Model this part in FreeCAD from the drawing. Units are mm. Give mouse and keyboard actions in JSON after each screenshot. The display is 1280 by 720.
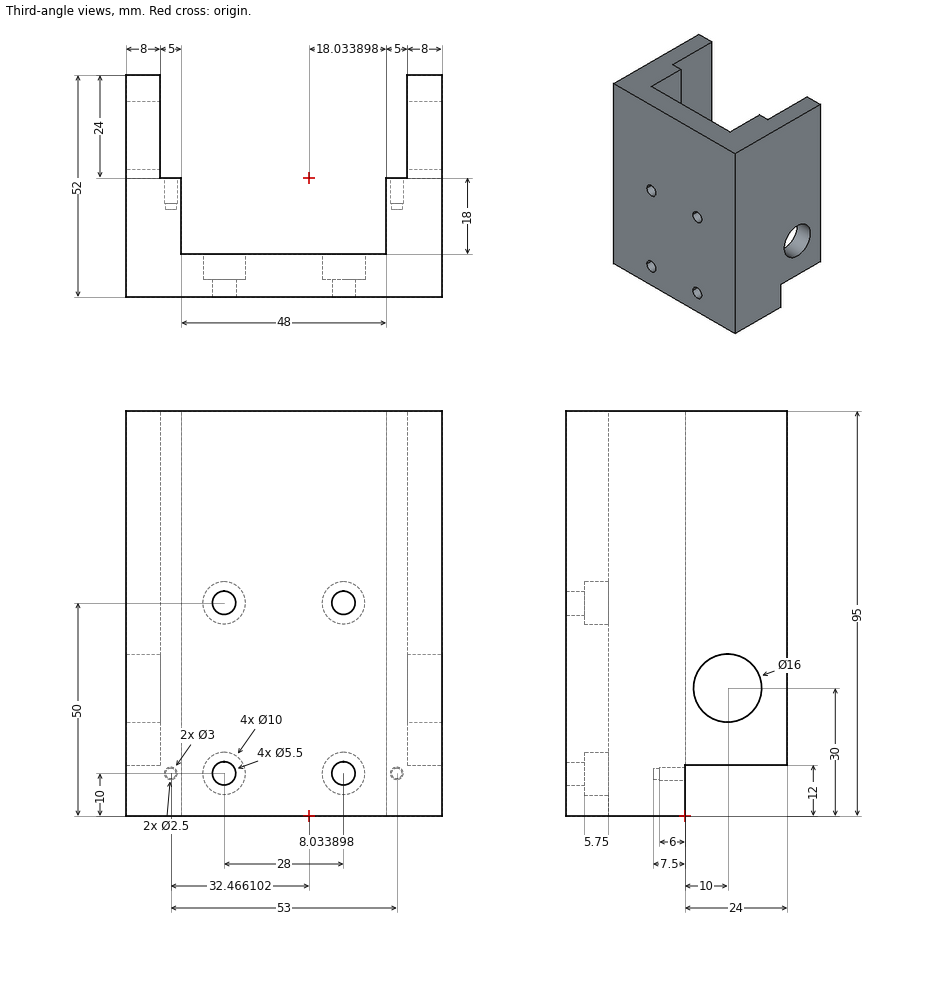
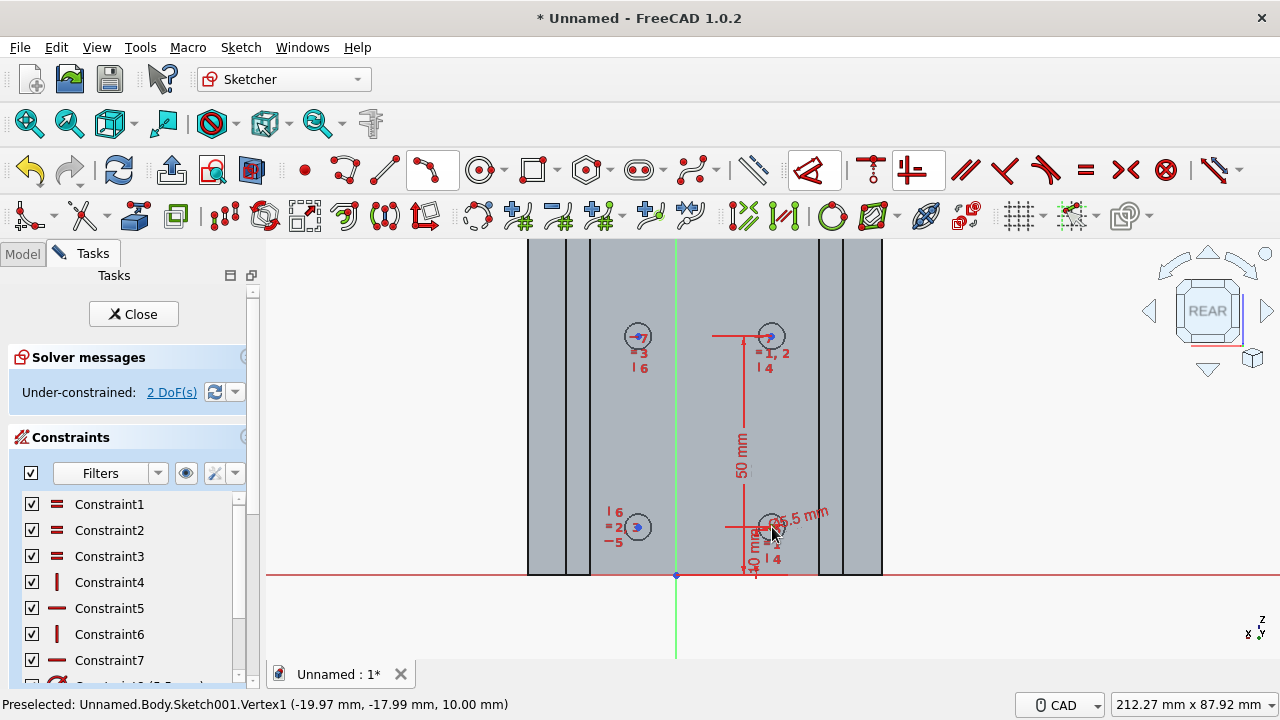
{"action": "left_click", "coordinate": [638, 527]}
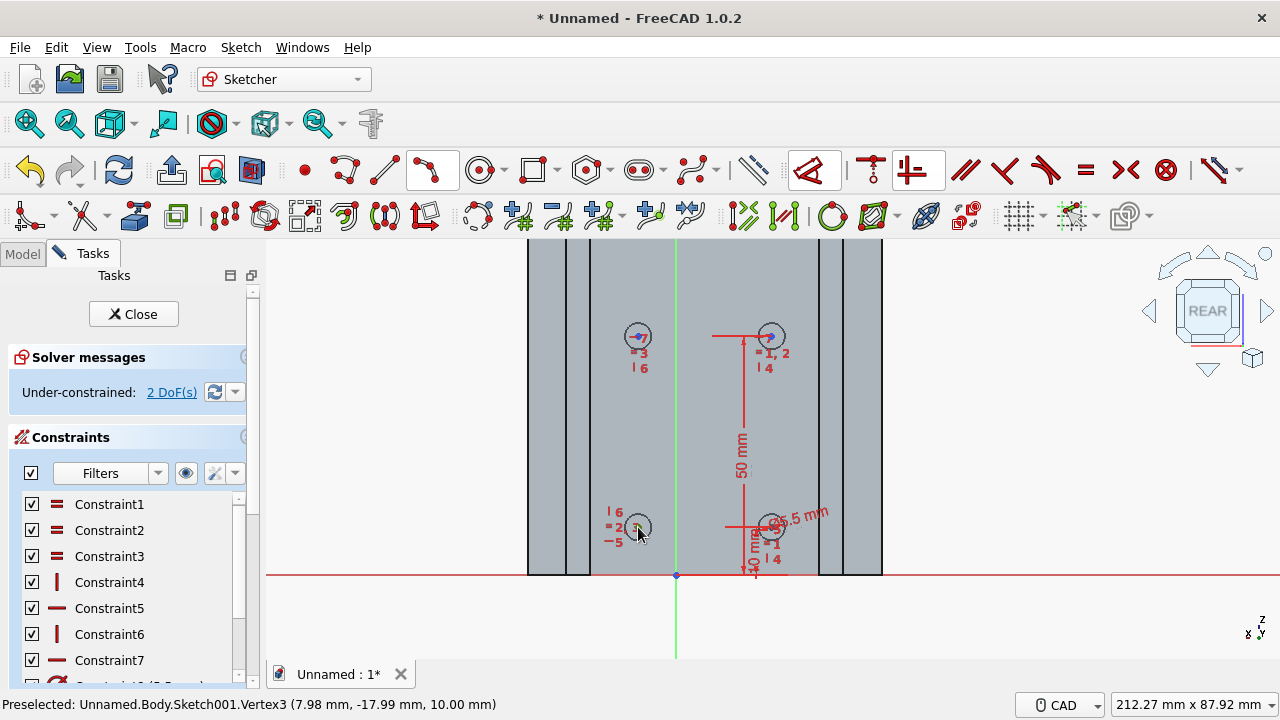
{"action": "key", "text": "l"}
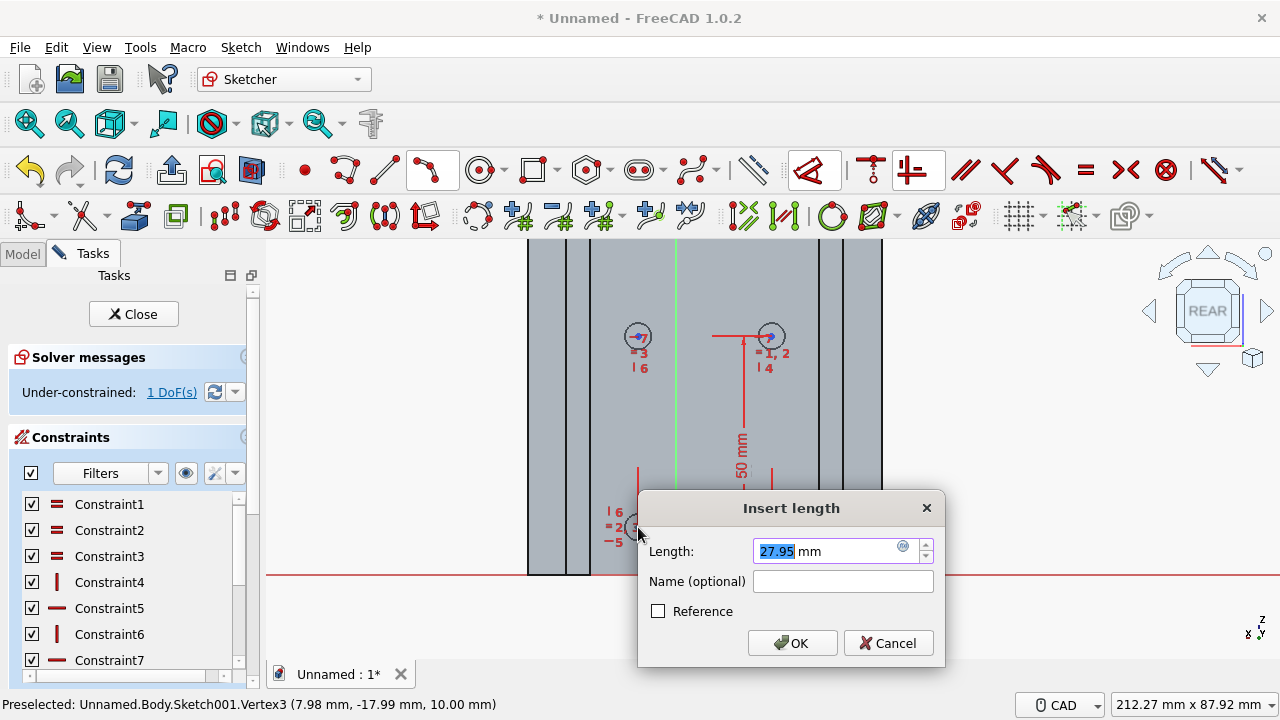
{"action": "type", "text": "28"}
{"action": "key", "text": "Return"}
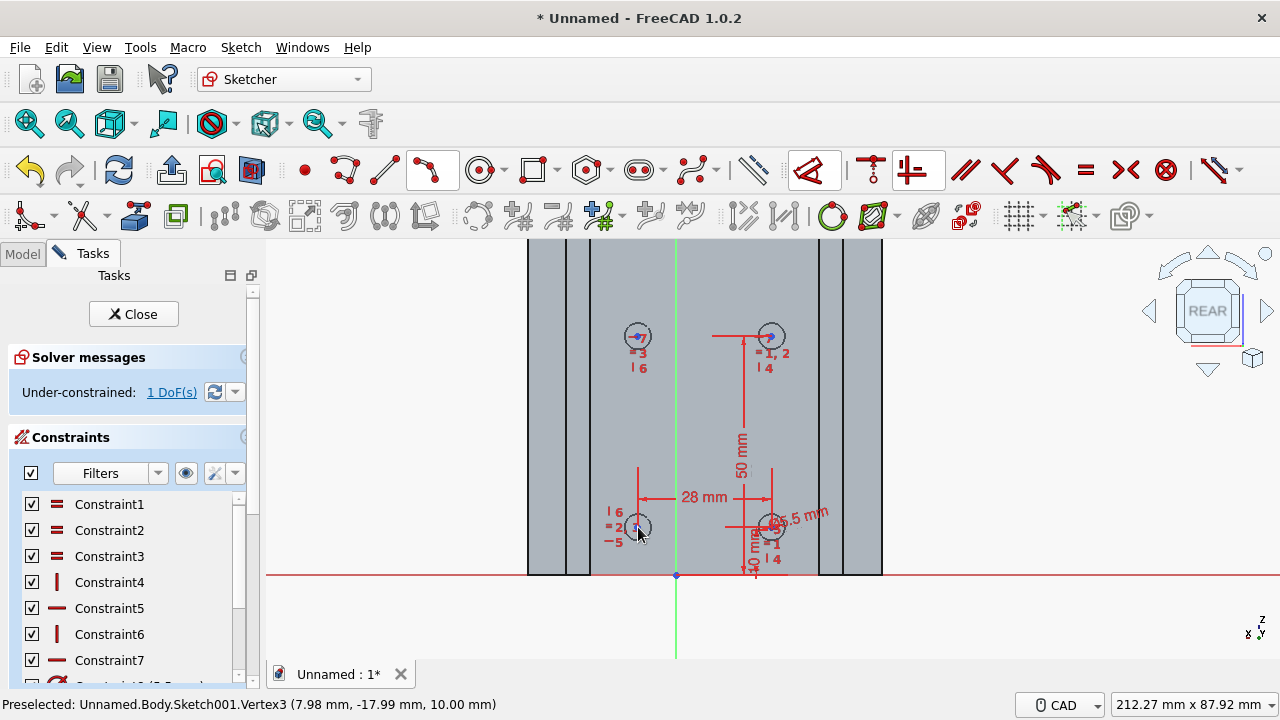
{"action": "left_click", "coordinate": [638, 527]}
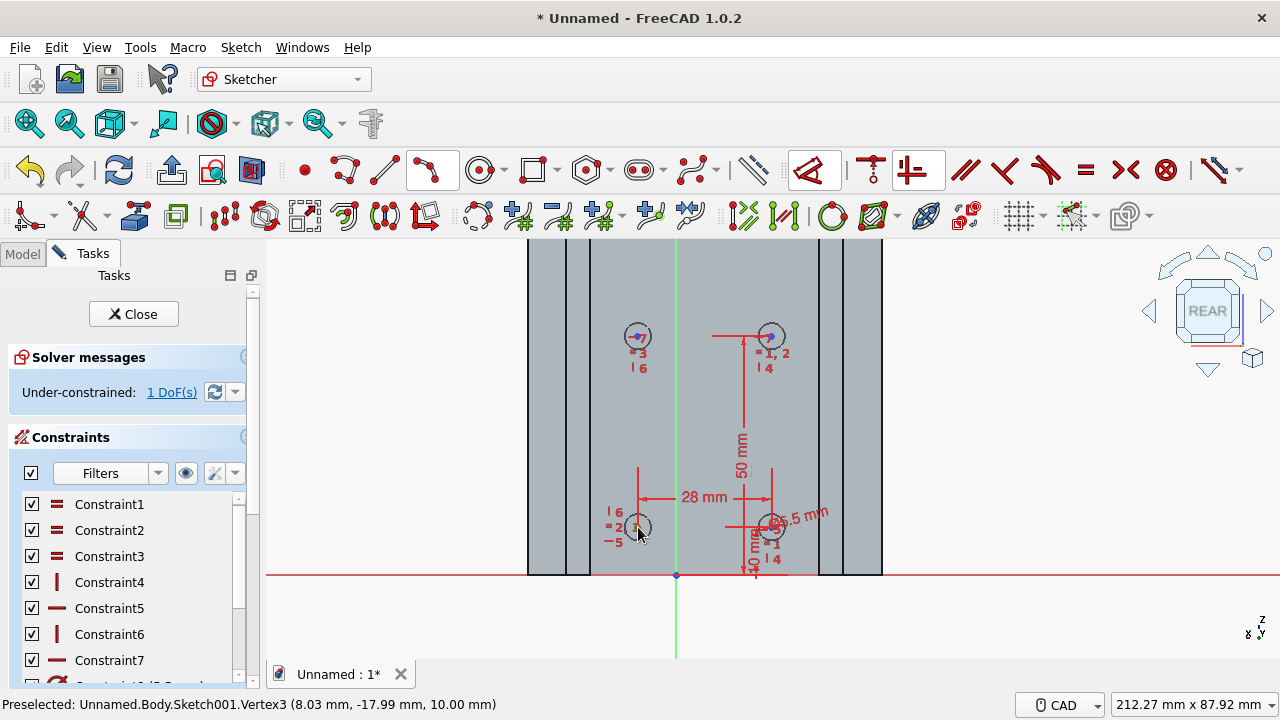
{"action": "key", "text": "l"}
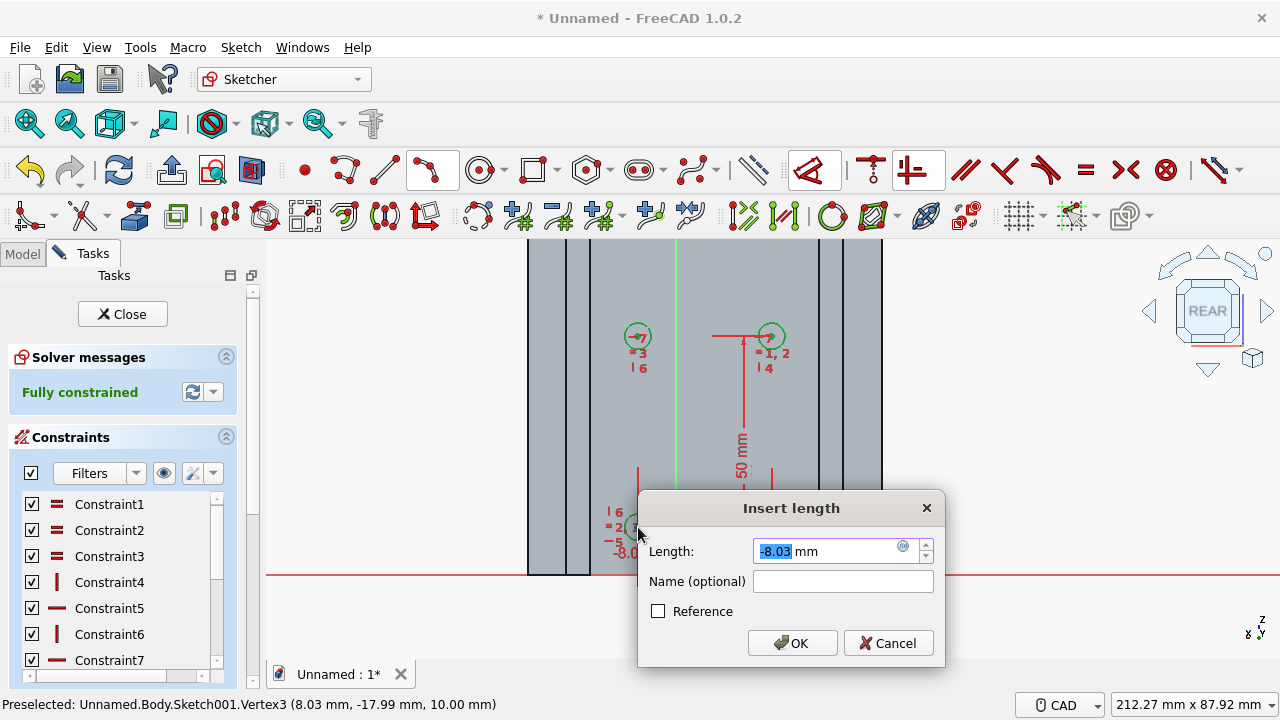
{"action": "type", "text": "-8.033898"}
{"action": "key", "text": "Return"}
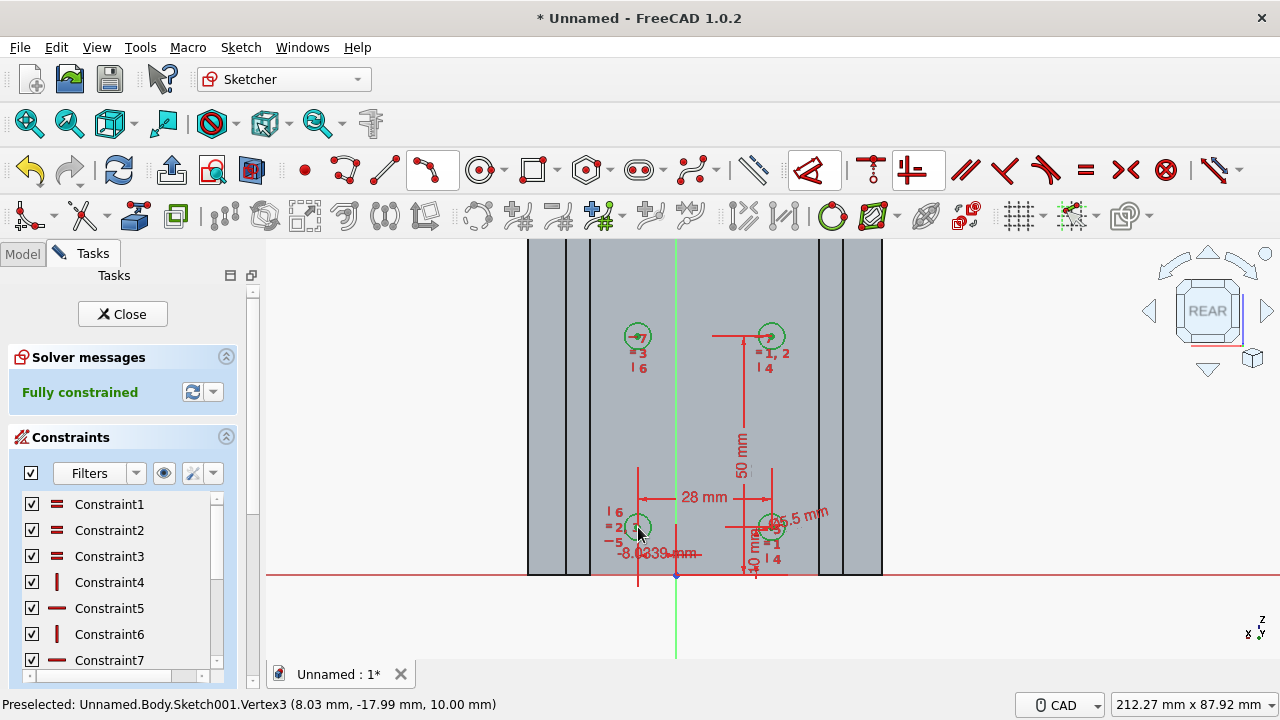
{"action": "left_click", "coordinate": [123, 314]}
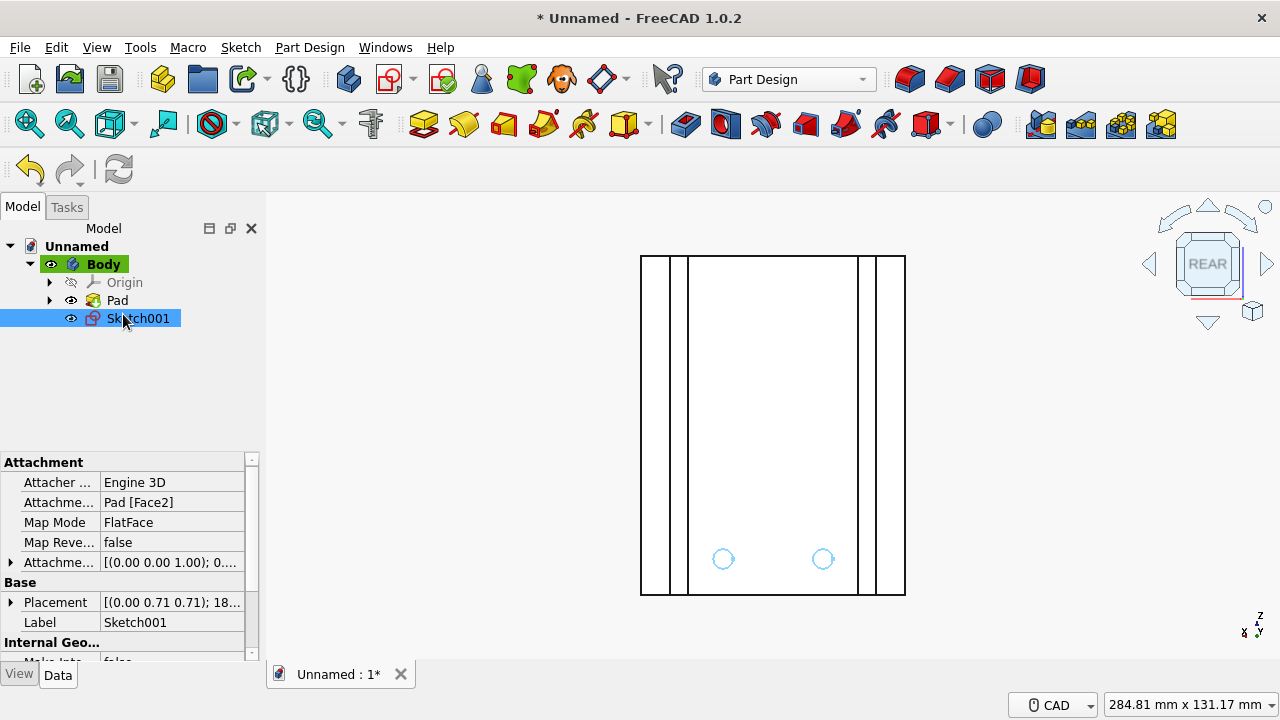
{"action": "left_click", "coordinate": [686, 124]}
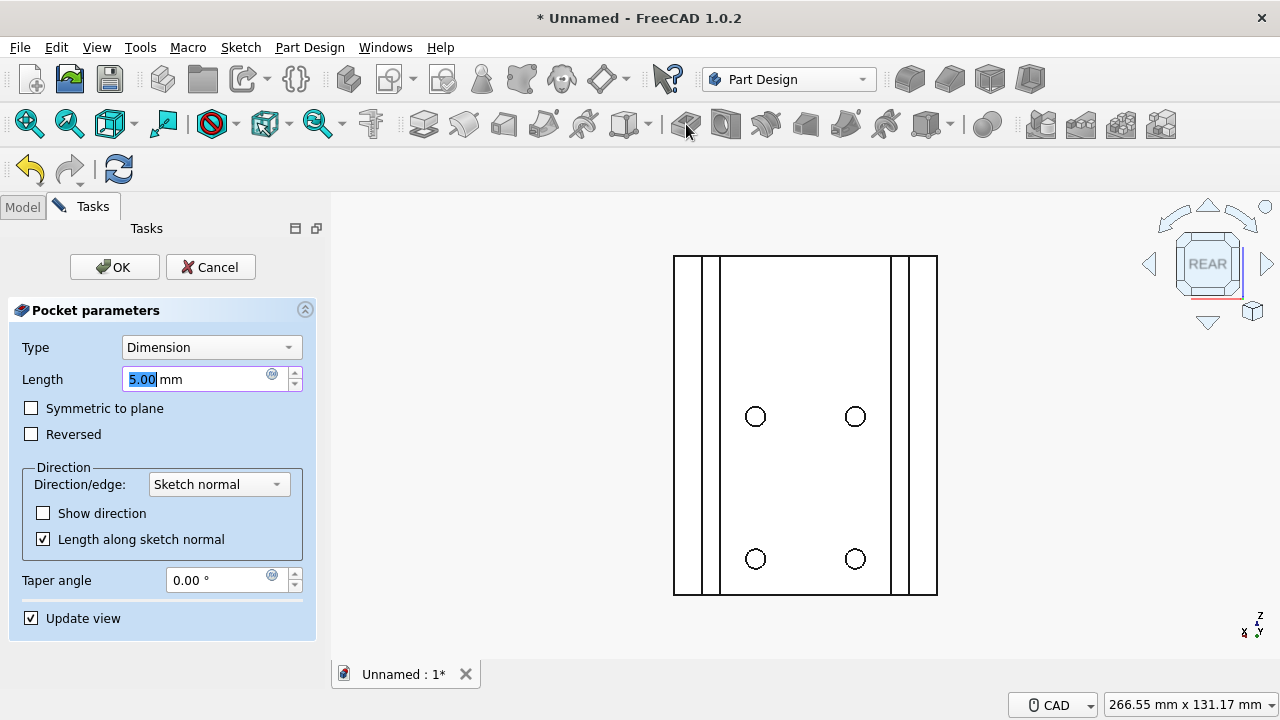
{"action": "left_click", "coordinate": [212, 348]}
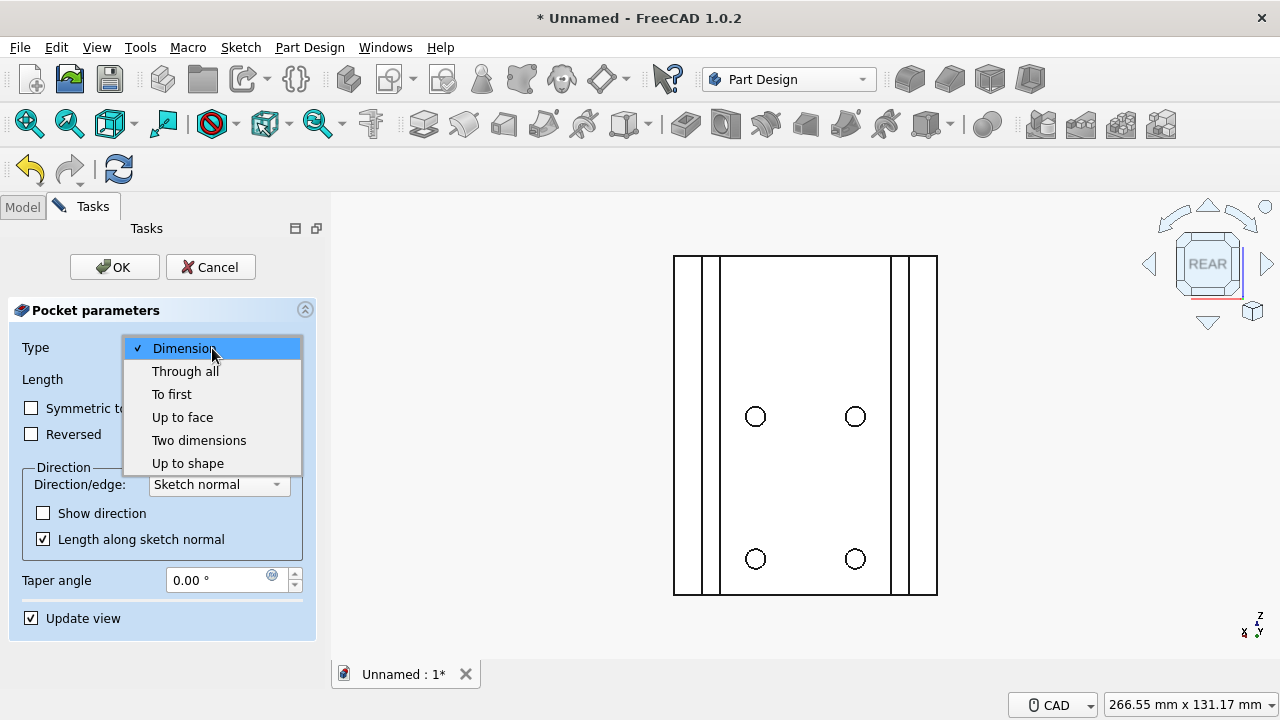
{"action": "left_click", "coordinate": [212, 372]}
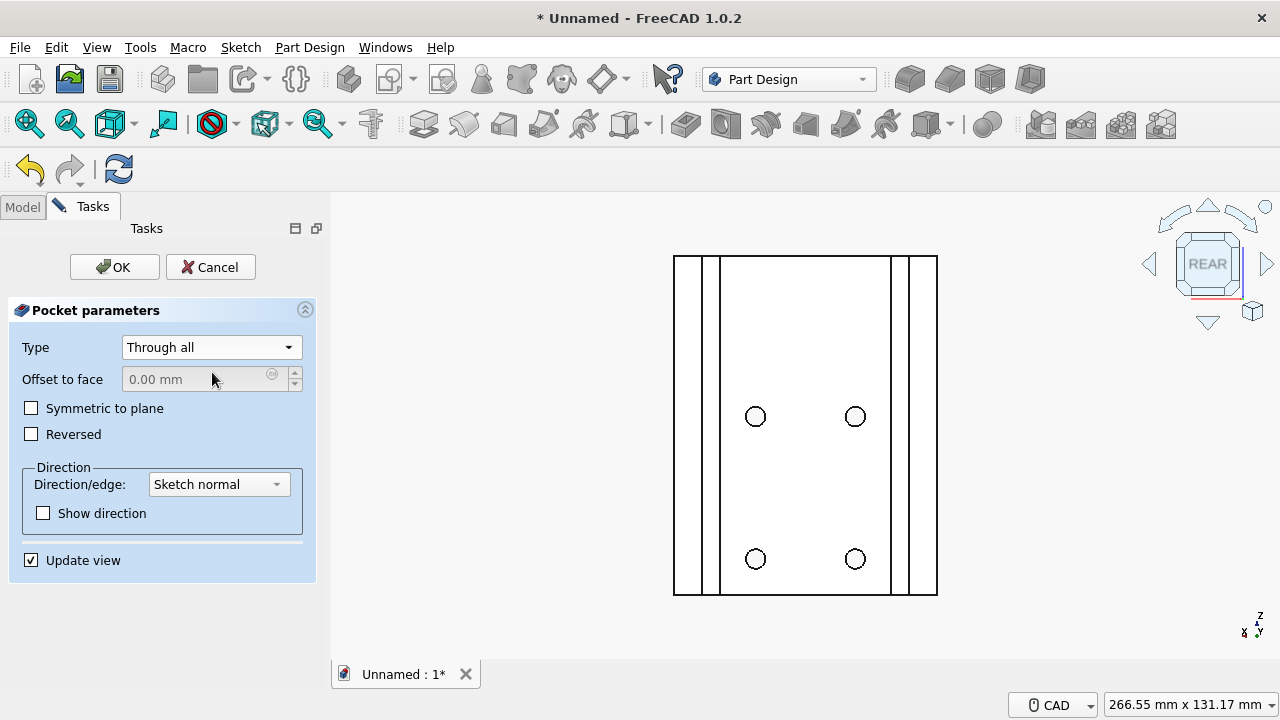
{"action": "left_click", "coordinate": [115, 267]}